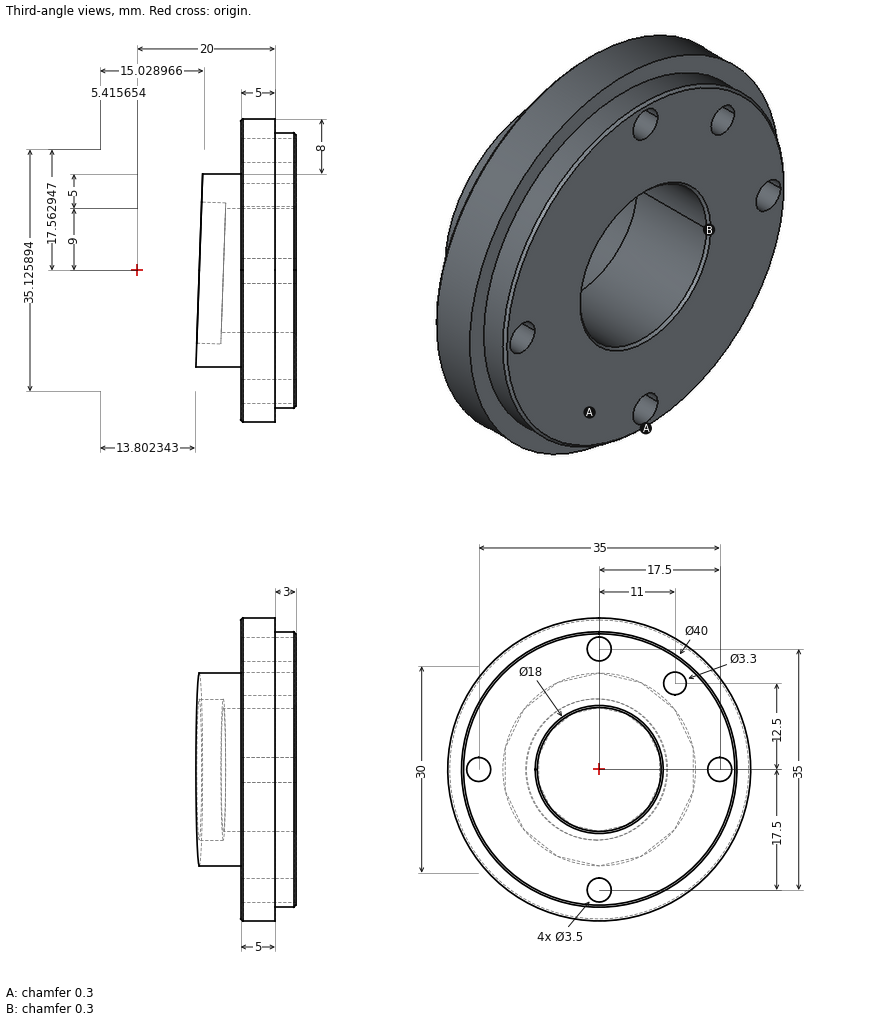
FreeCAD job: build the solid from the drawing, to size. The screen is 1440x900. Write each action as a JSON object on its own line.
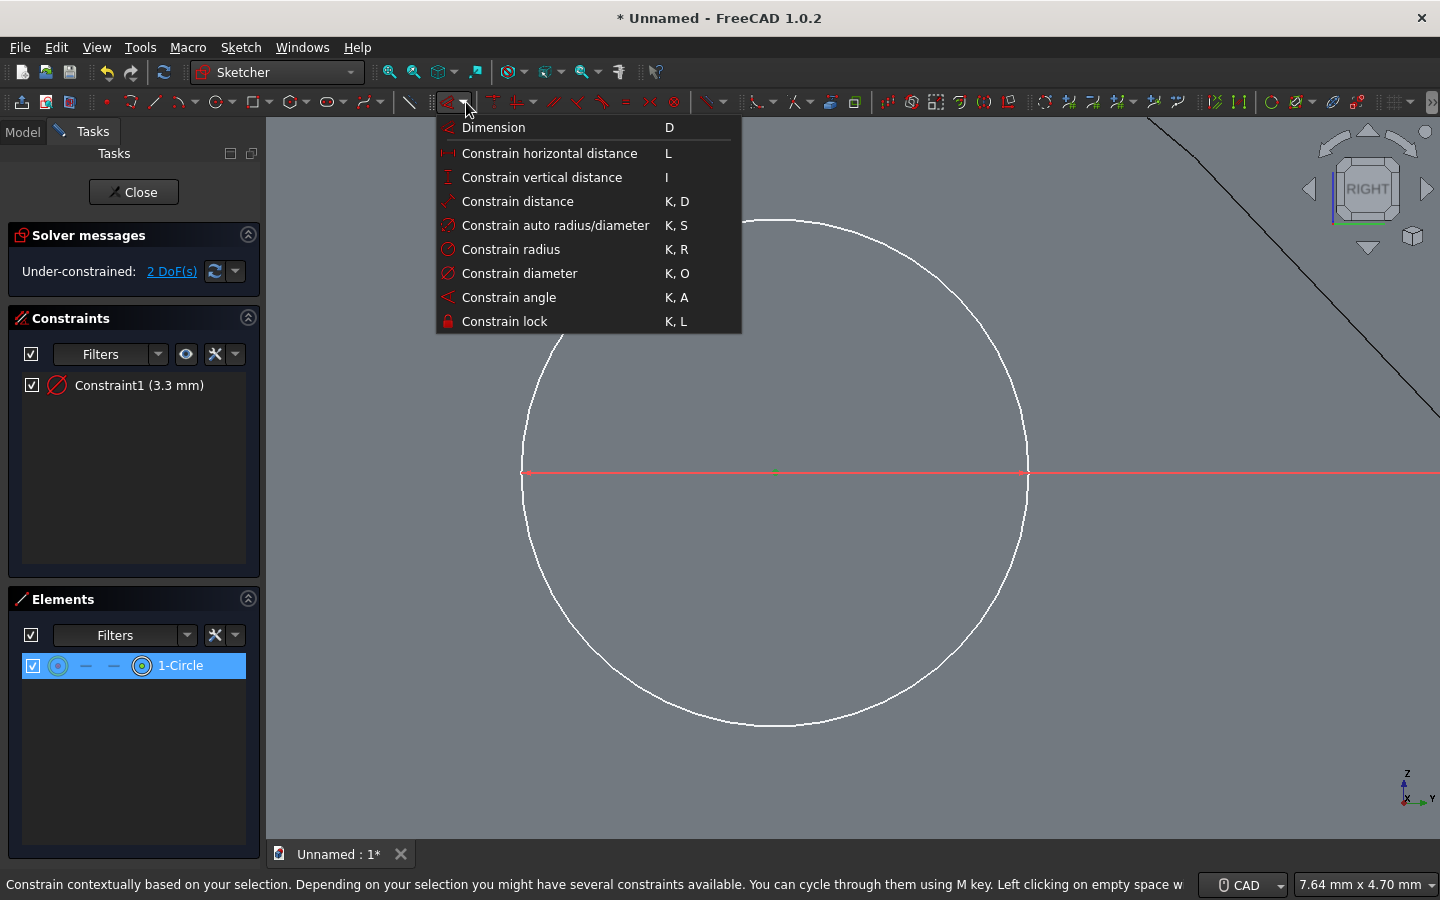
{"action": "left_click", "coordinate": [589, 153]}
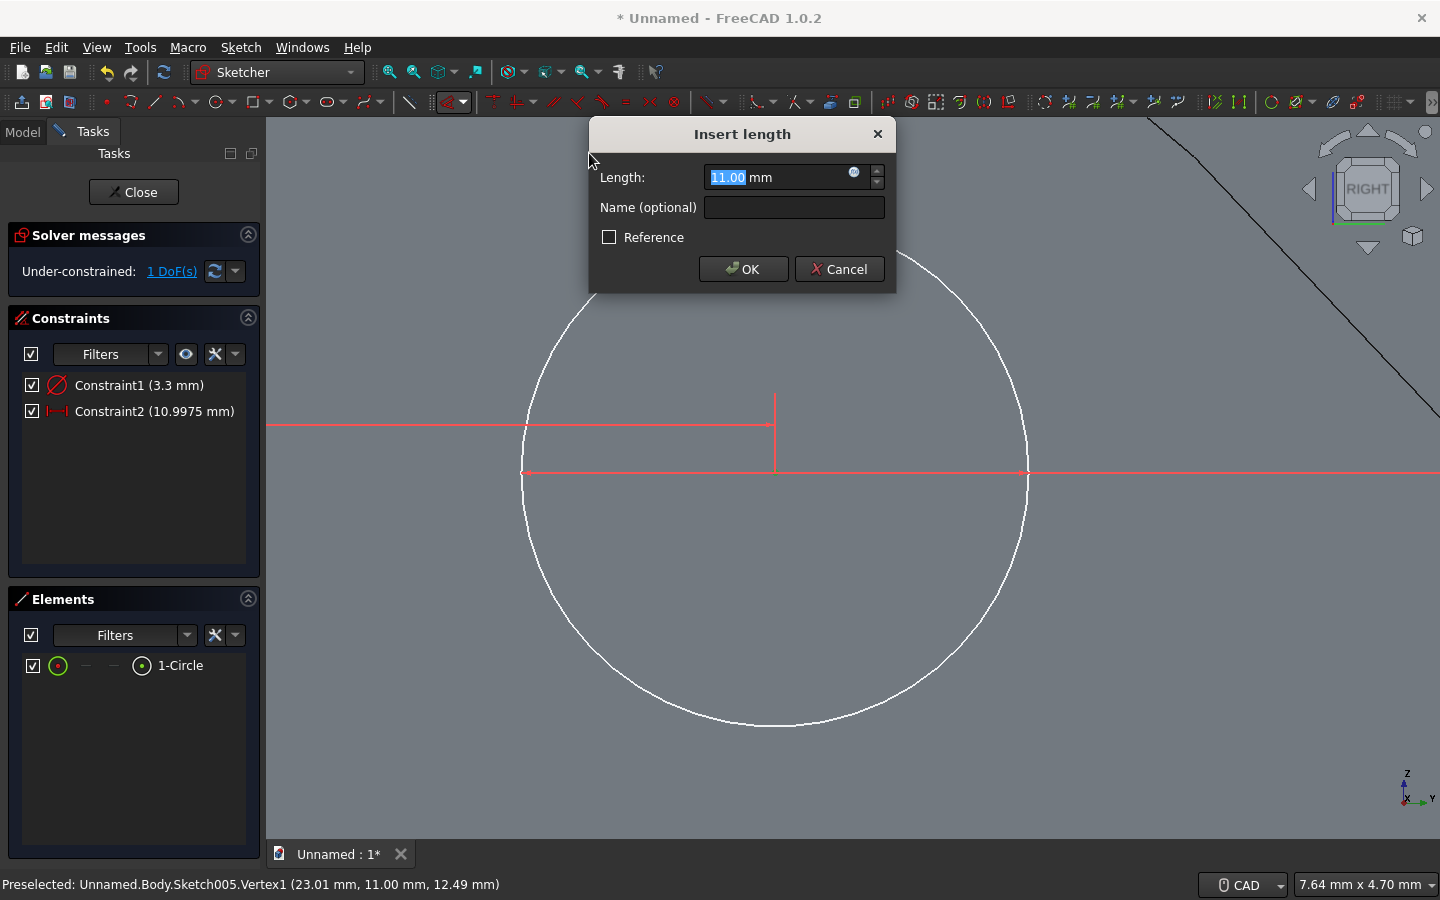
{"action": "type", "text": "11"}
{"action": "key", "text": "Return"}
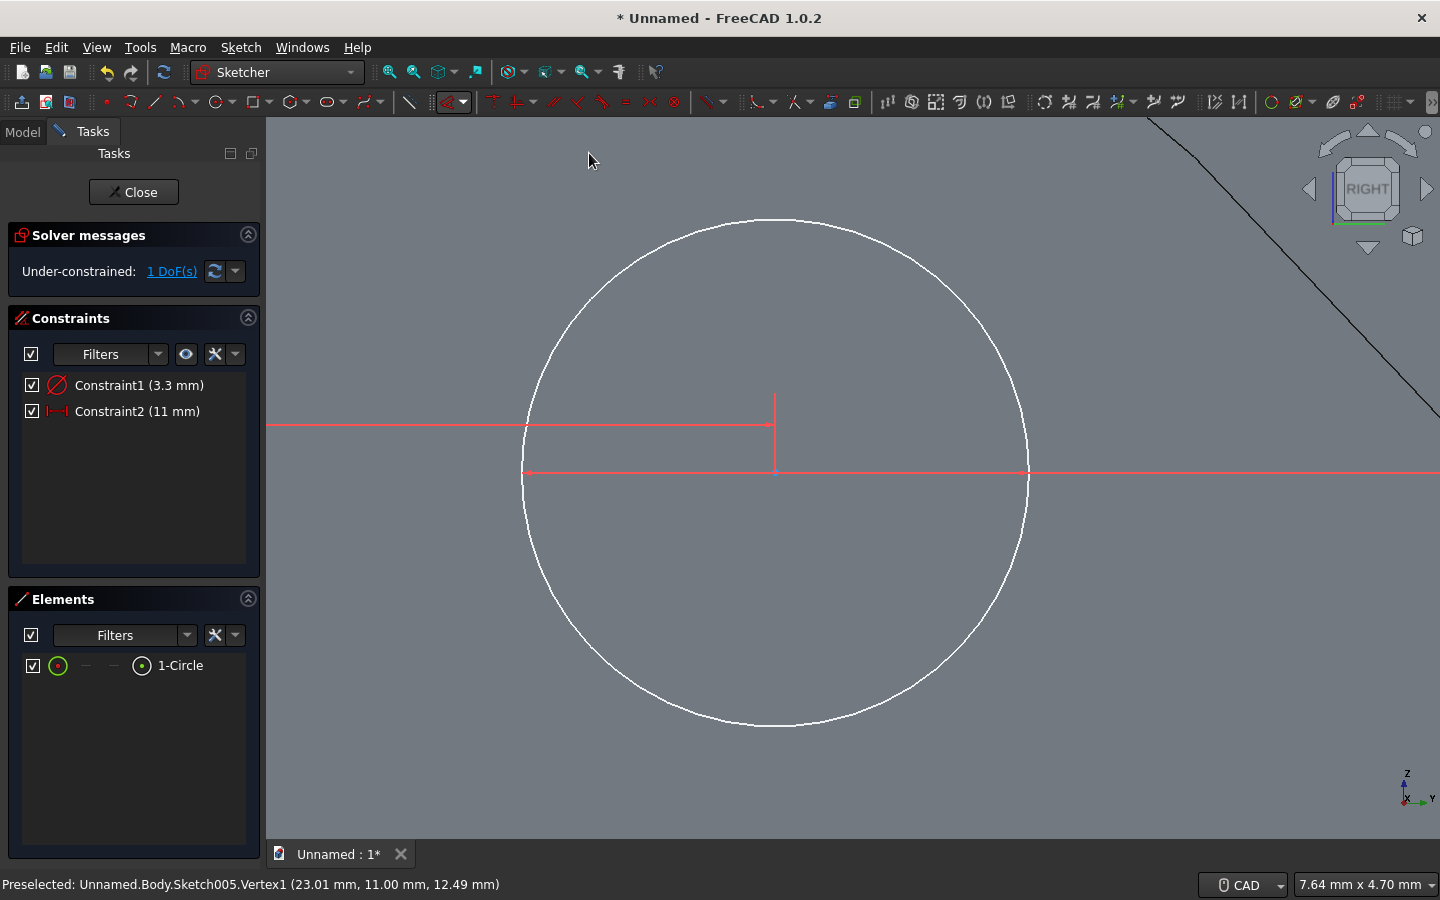
{"action": "left_click", "coordinate": [775, 473]}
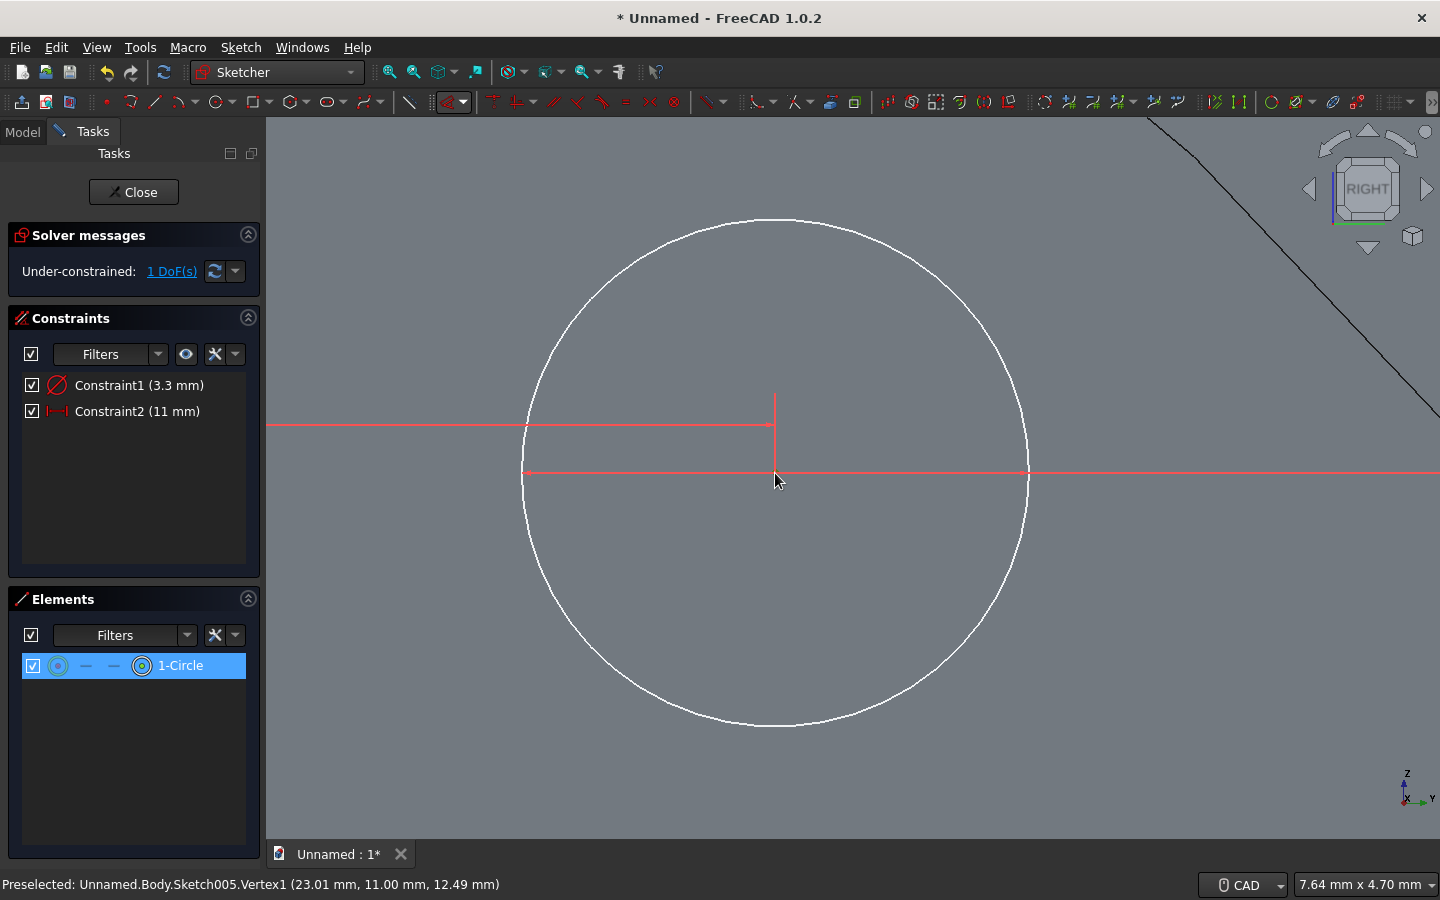
{"action": "key", "text": "i"}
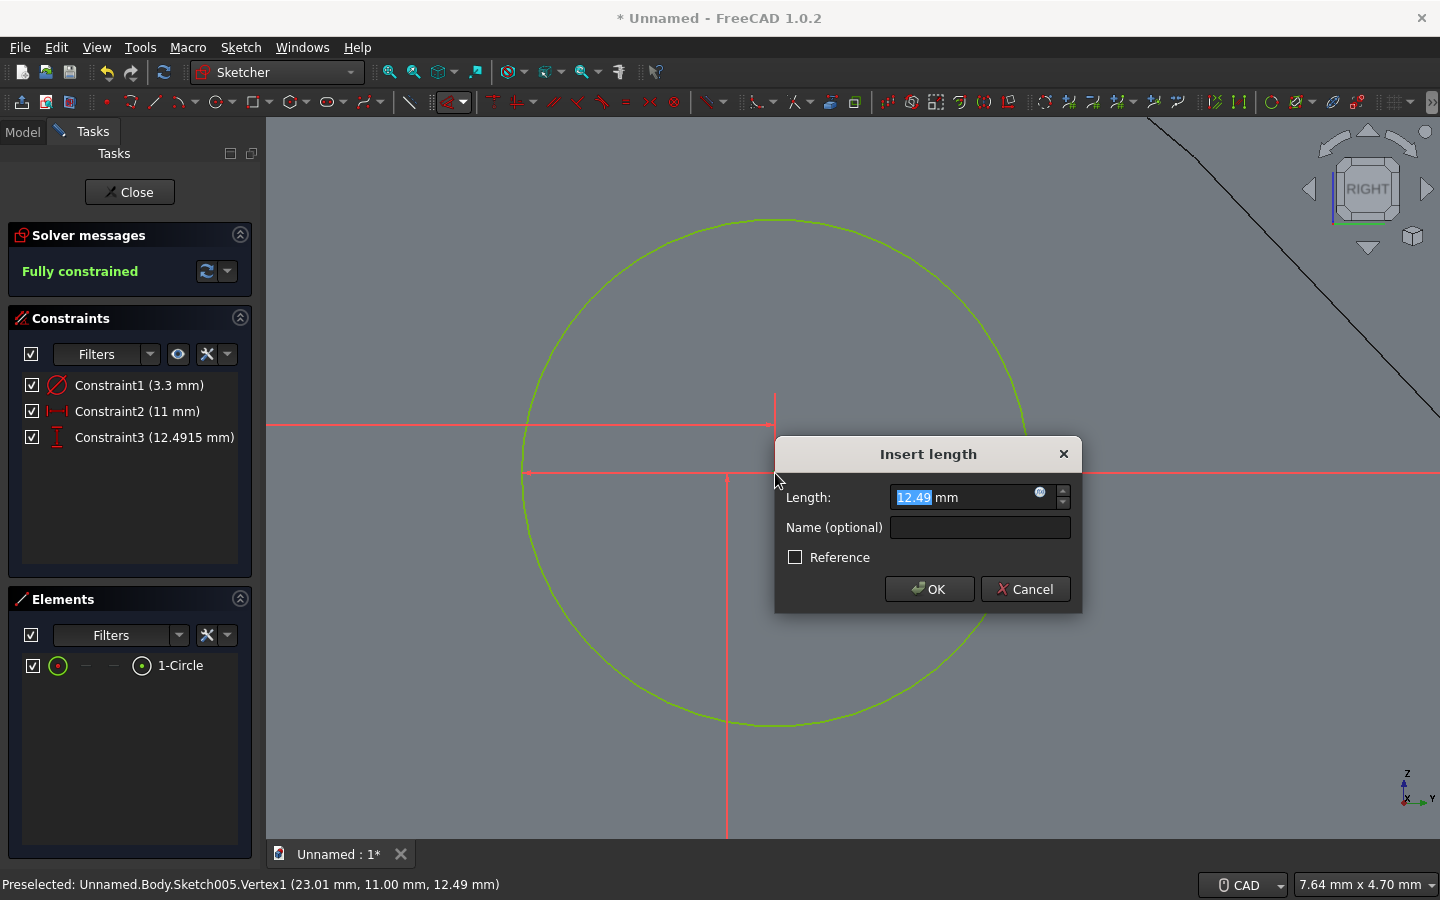
{"action": "type", "text": "12.5"}
{"action": "key", "text": "Return"}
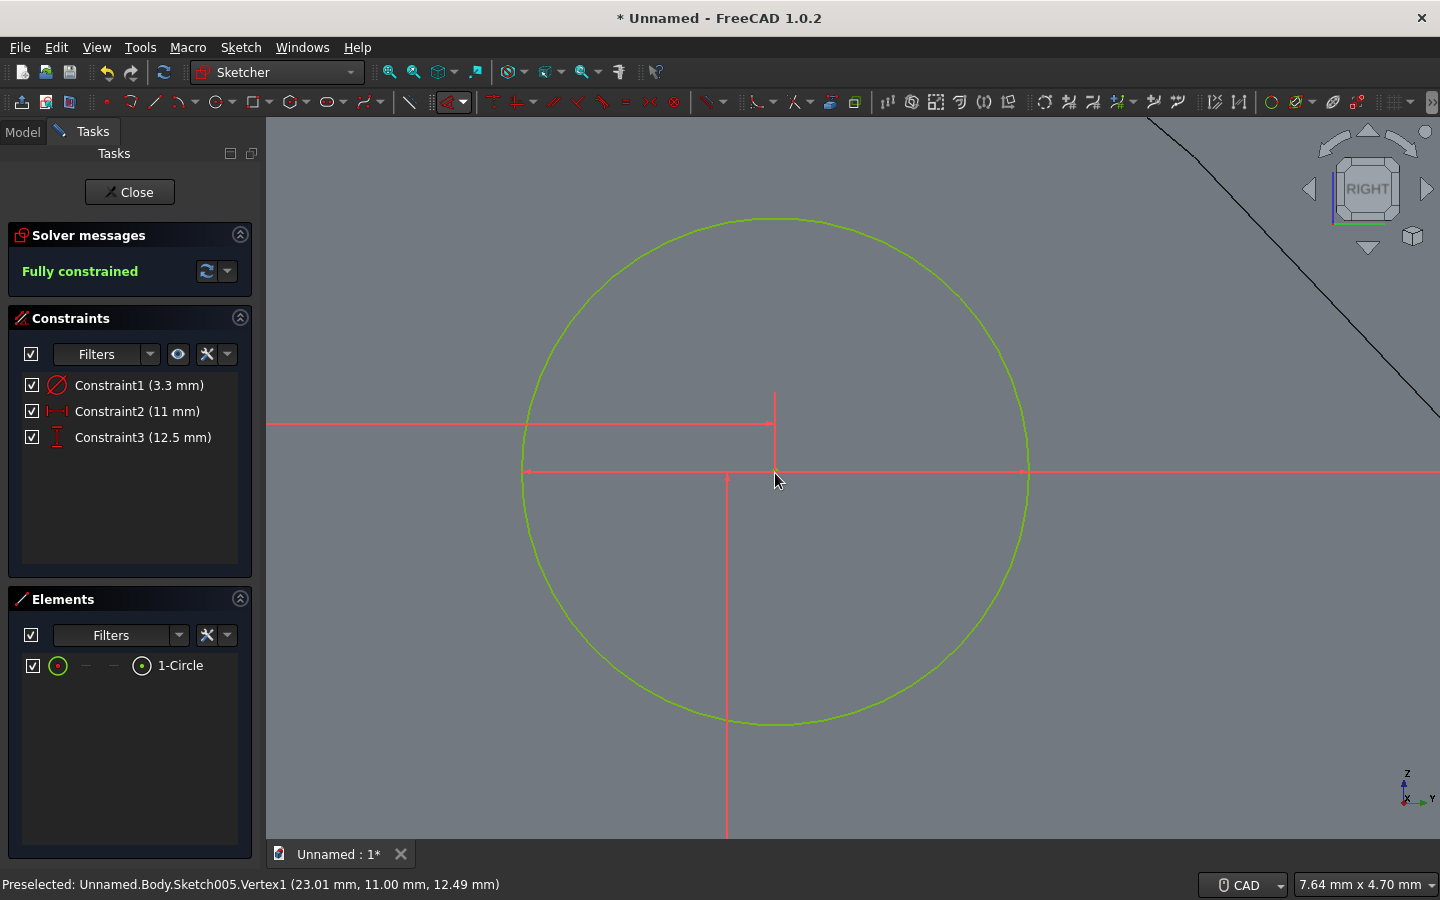
{"action": "left_click", "coordinate": [130, 192]}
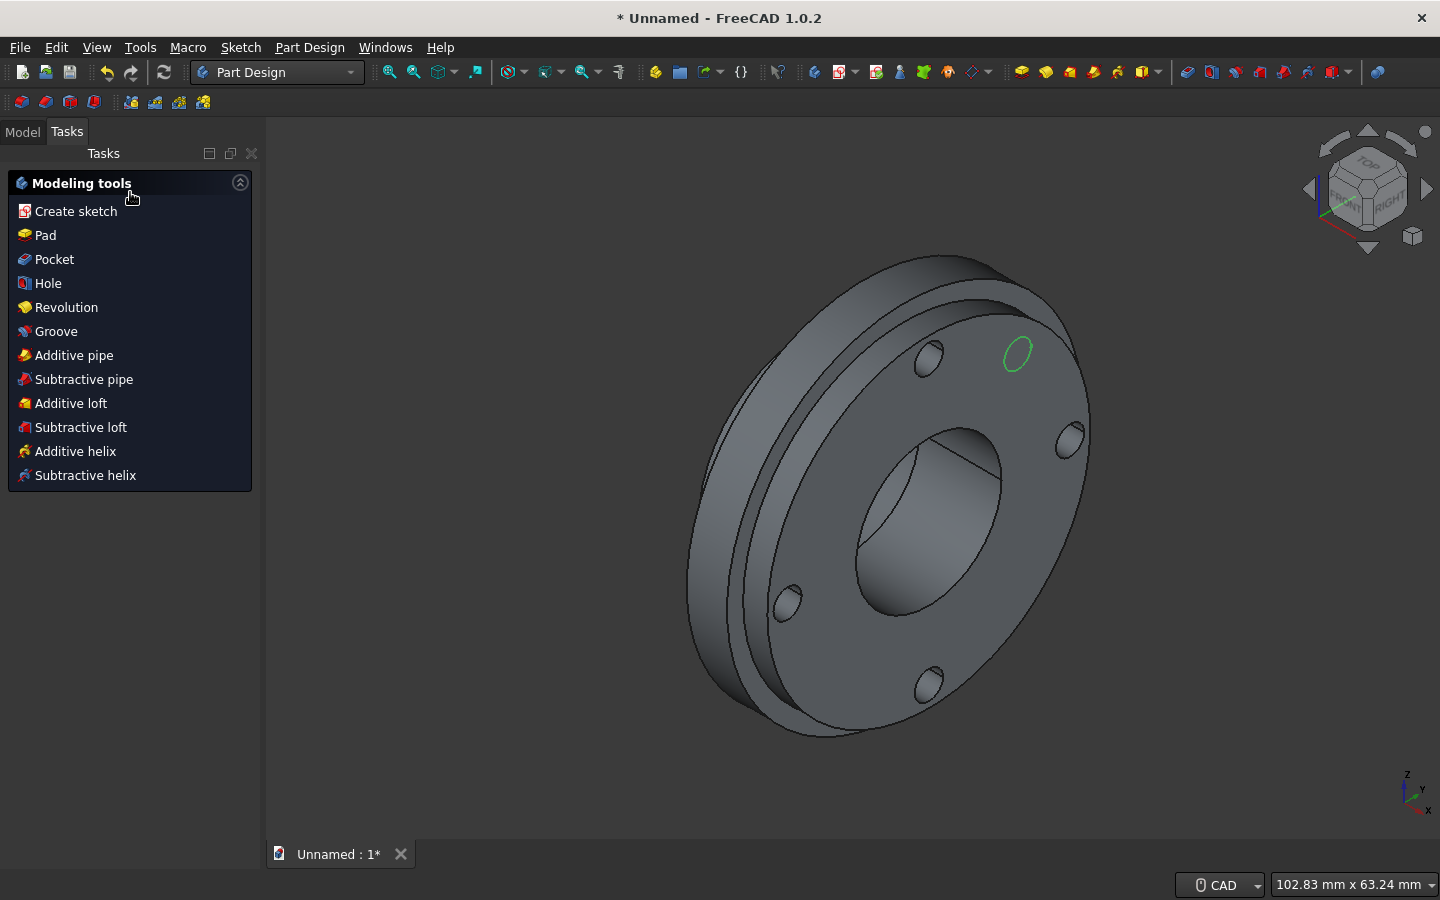
{"action": "left_click", "coordinate": [1188, 72]}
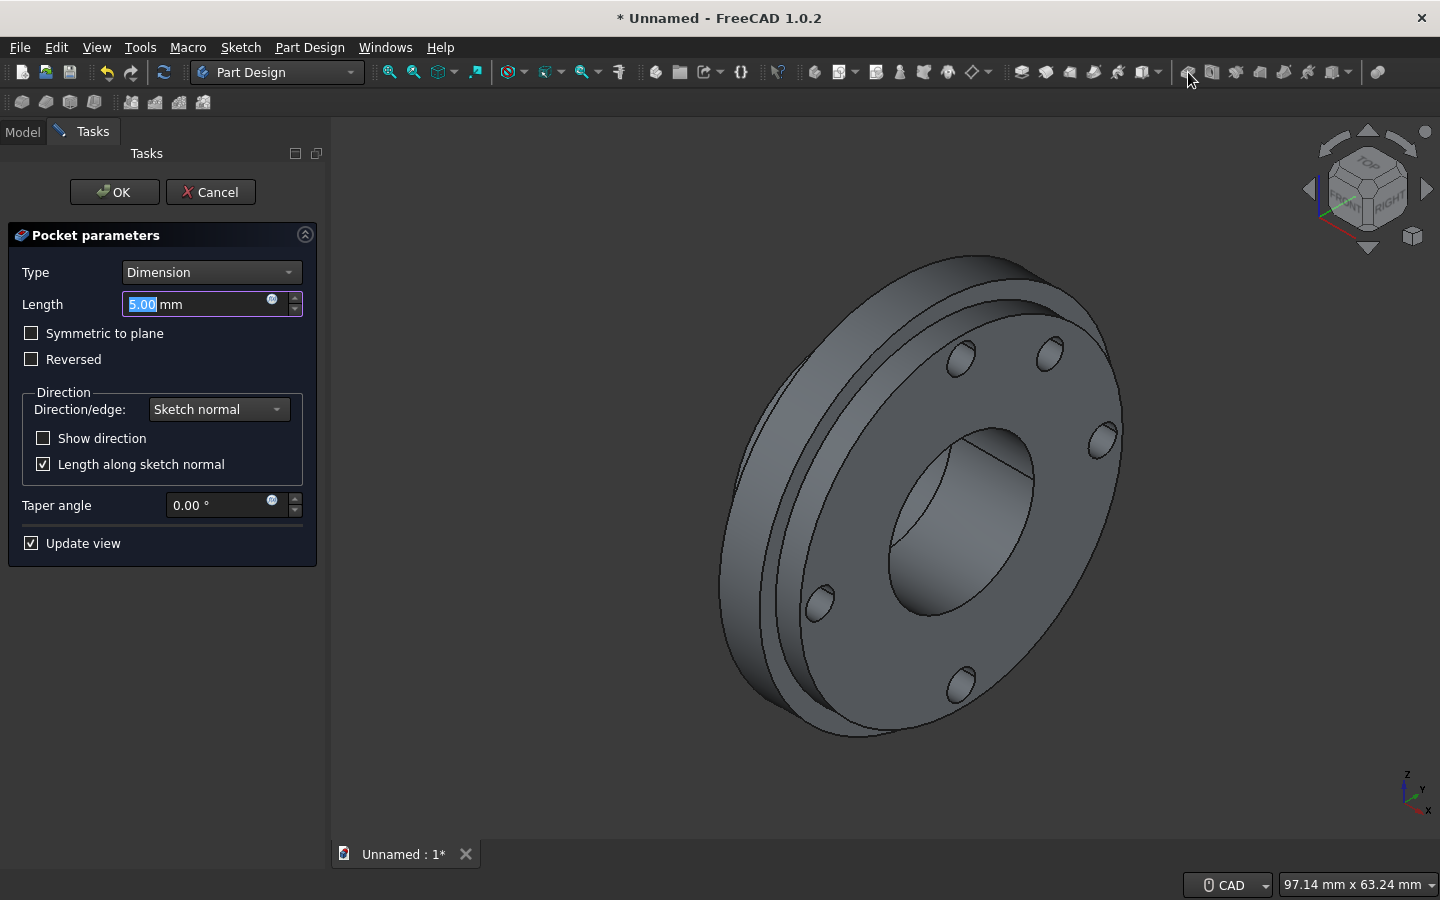
{"action": "left_click", "coordinate": [212, 272]}